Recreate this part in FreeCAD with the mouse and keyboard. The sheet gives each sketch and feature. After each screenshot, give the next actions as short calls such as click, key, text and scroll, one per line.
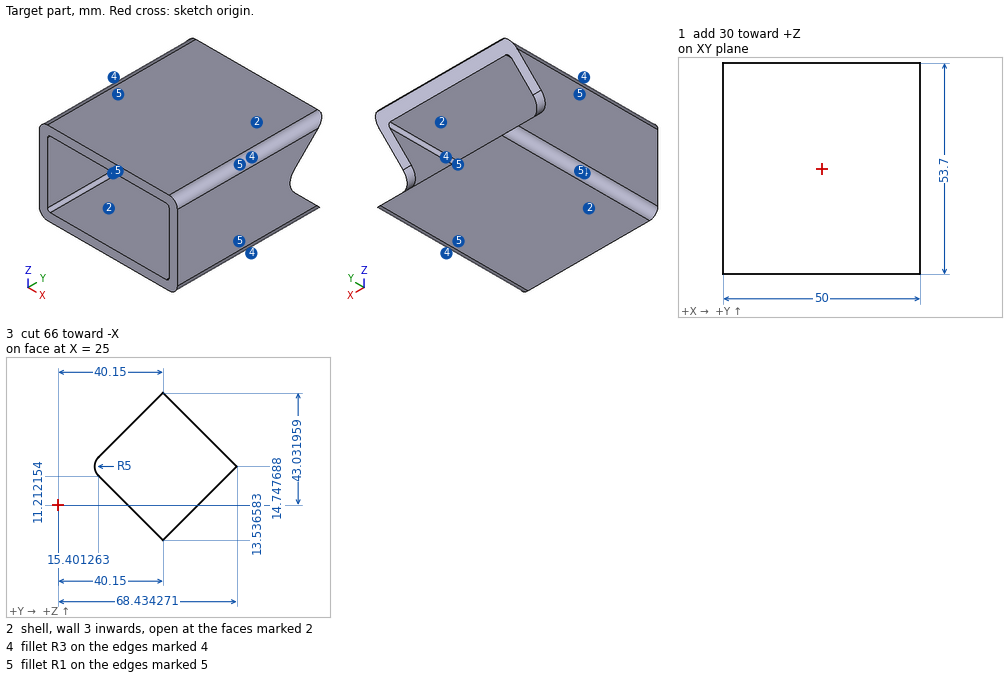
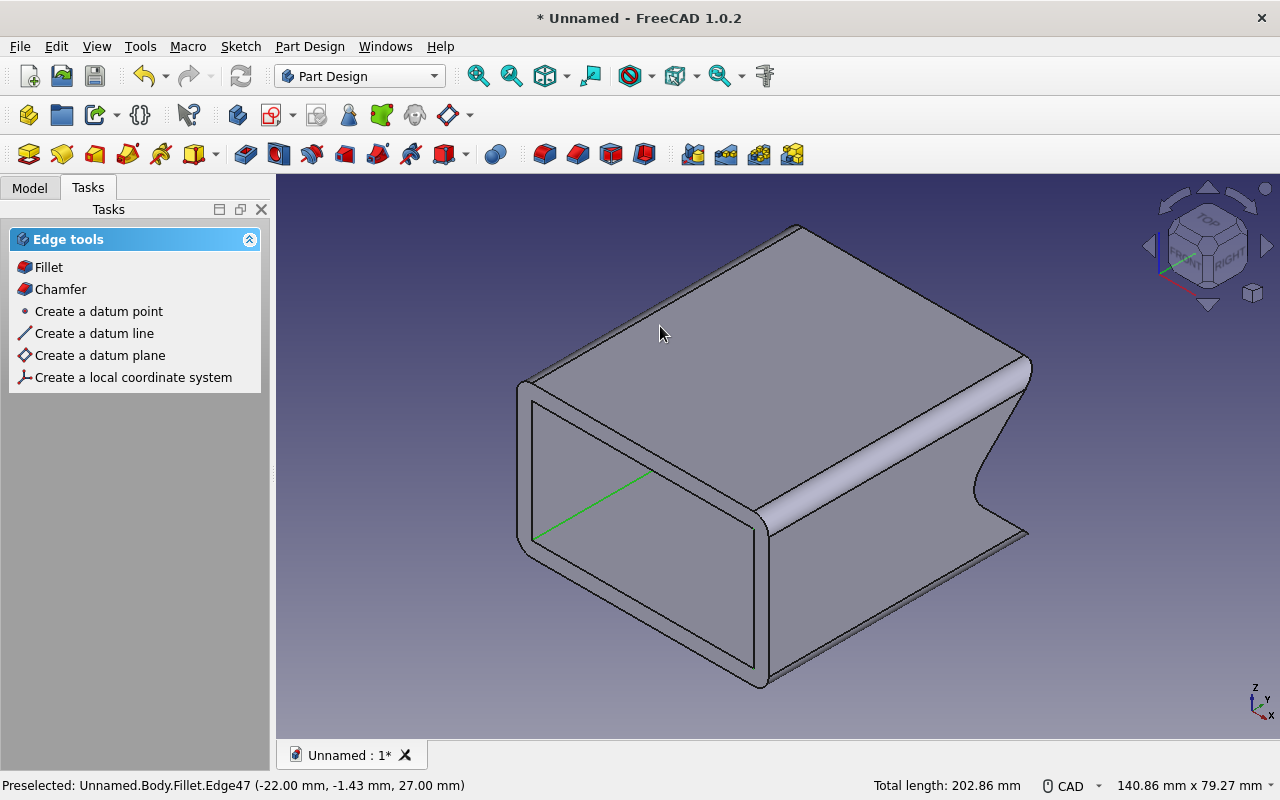
click(545, 154)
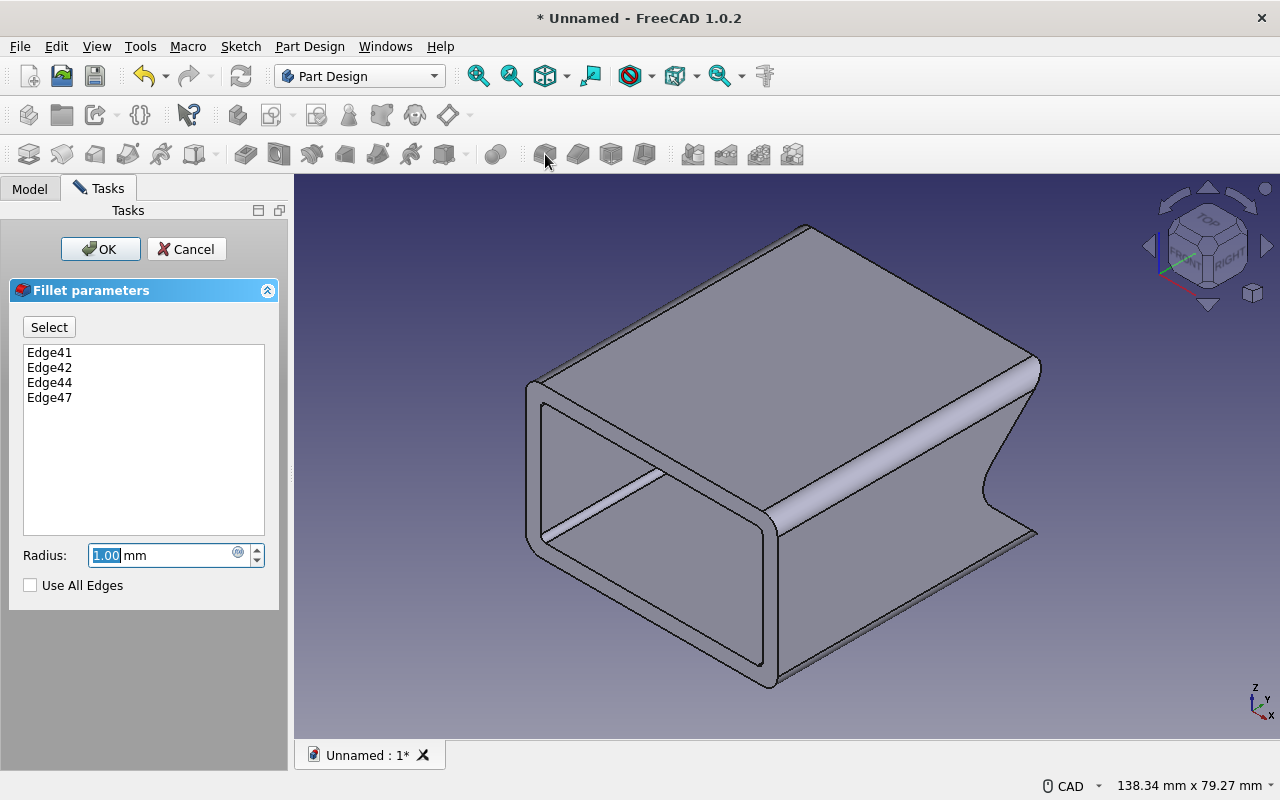
text(1)
key(Tab)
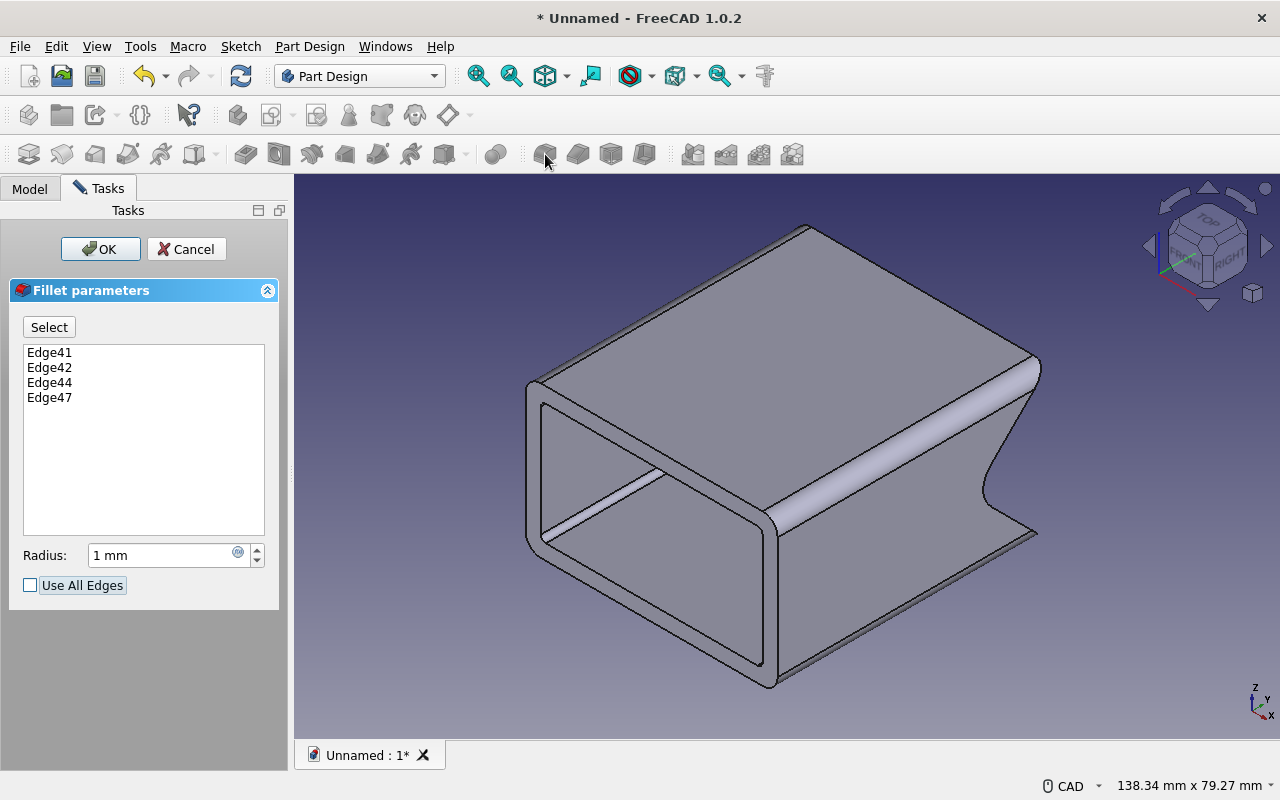
click(101, 249)